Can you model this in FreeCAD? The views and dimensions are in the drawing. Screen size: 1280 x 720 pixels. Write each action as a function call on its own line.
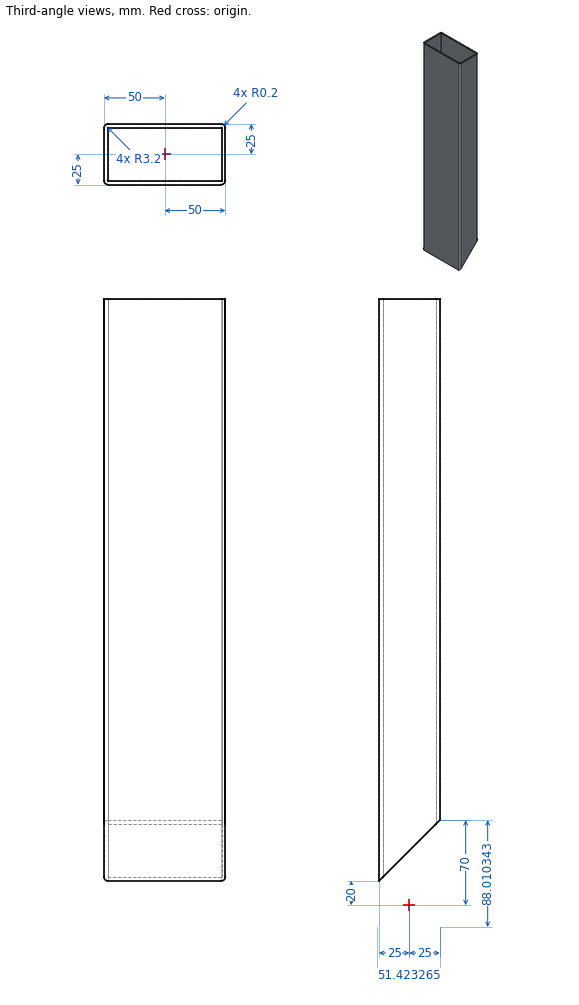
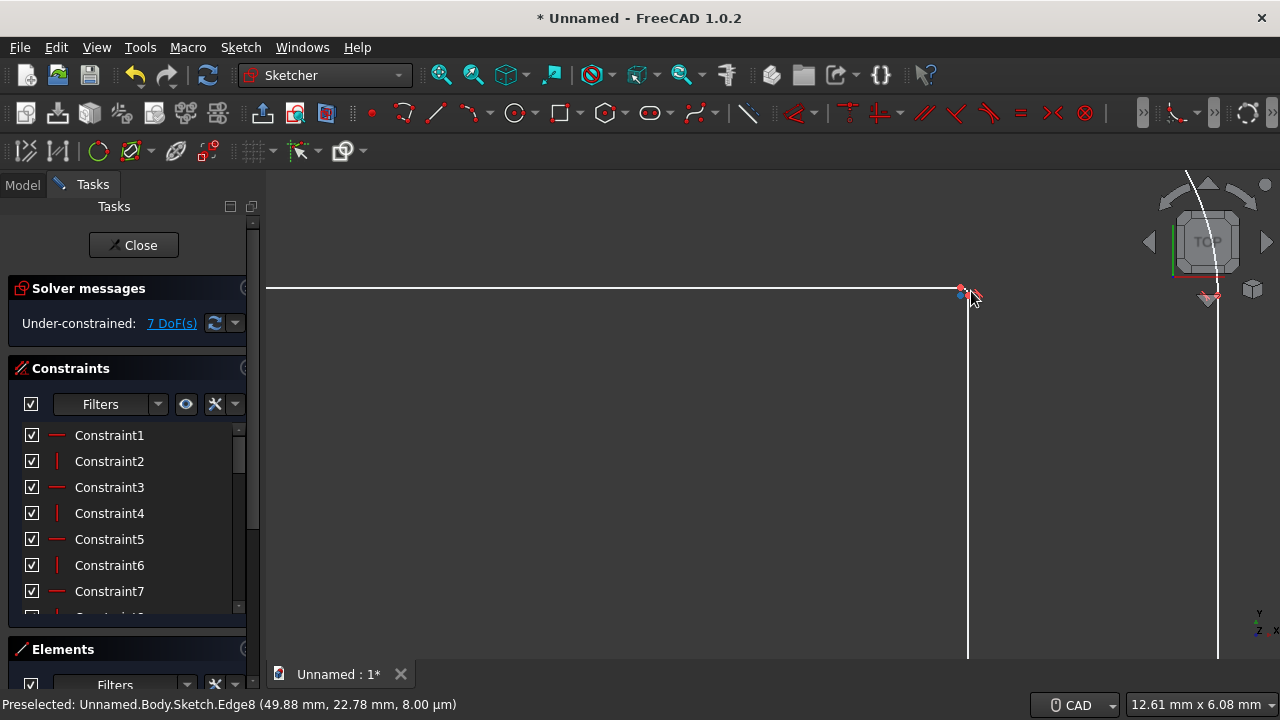
scroll(966, 290, up, 4)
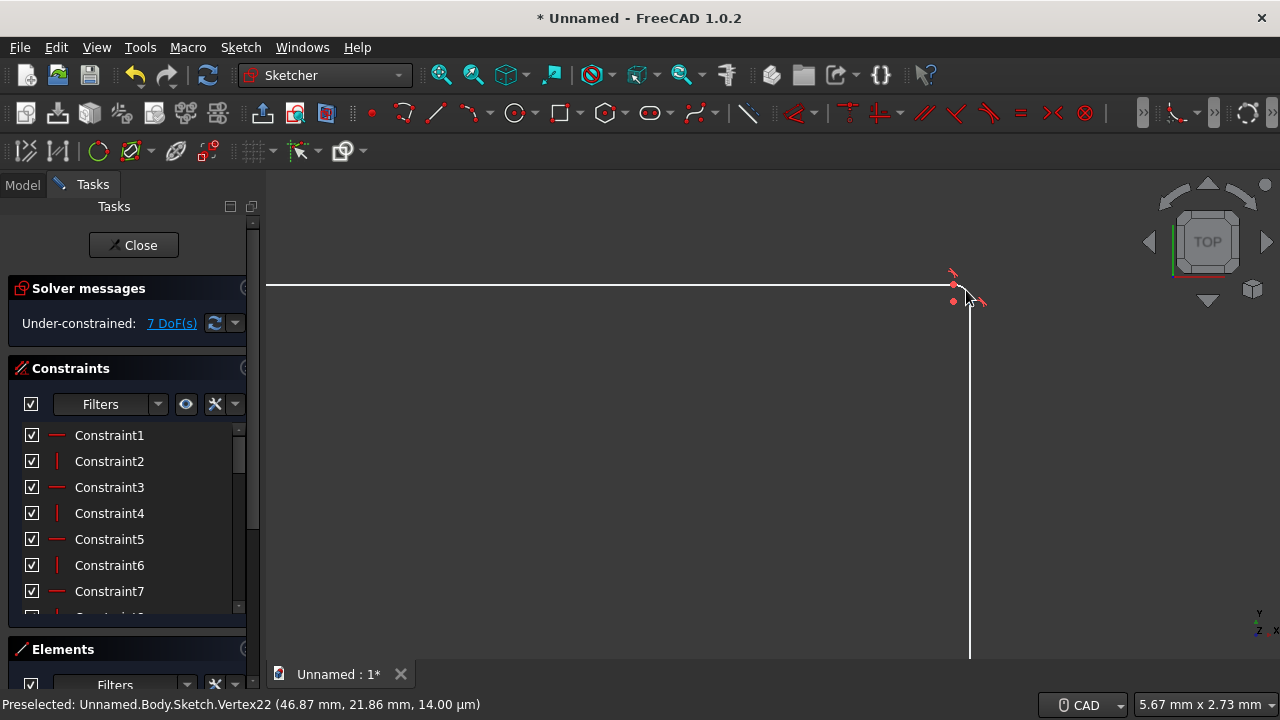
click(965, 290)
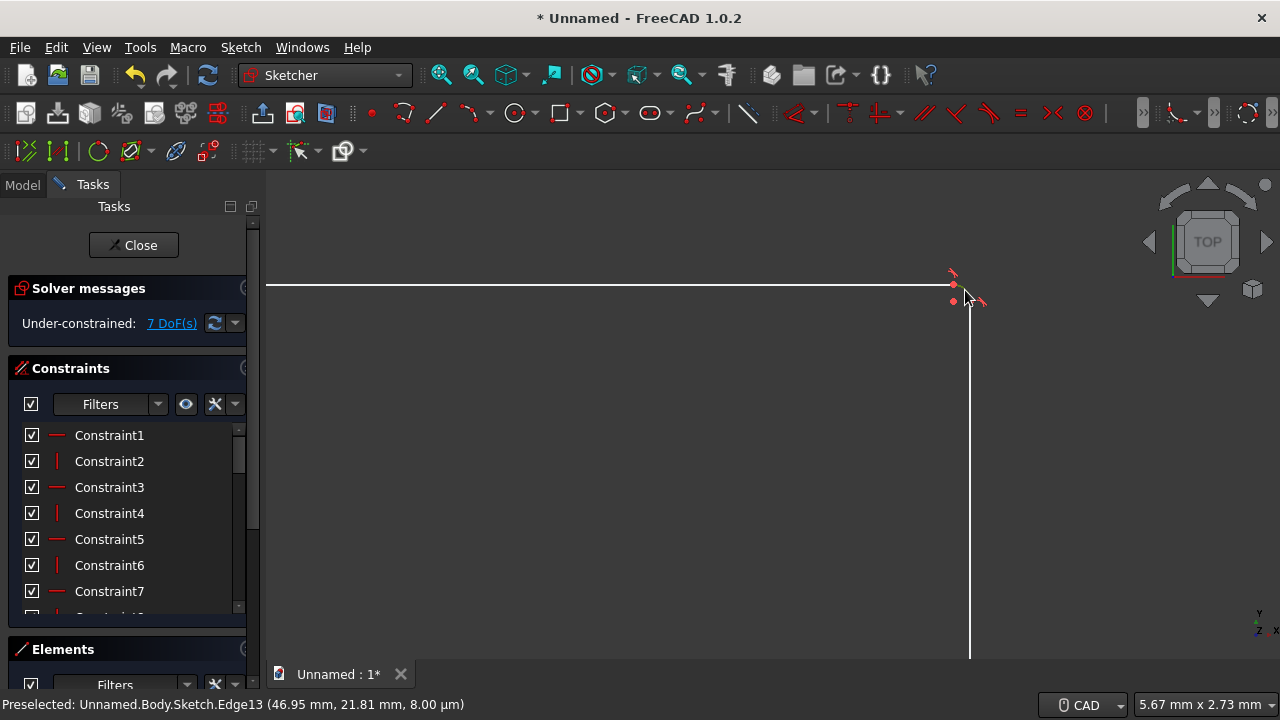
scroll(1050, 254, down, 16)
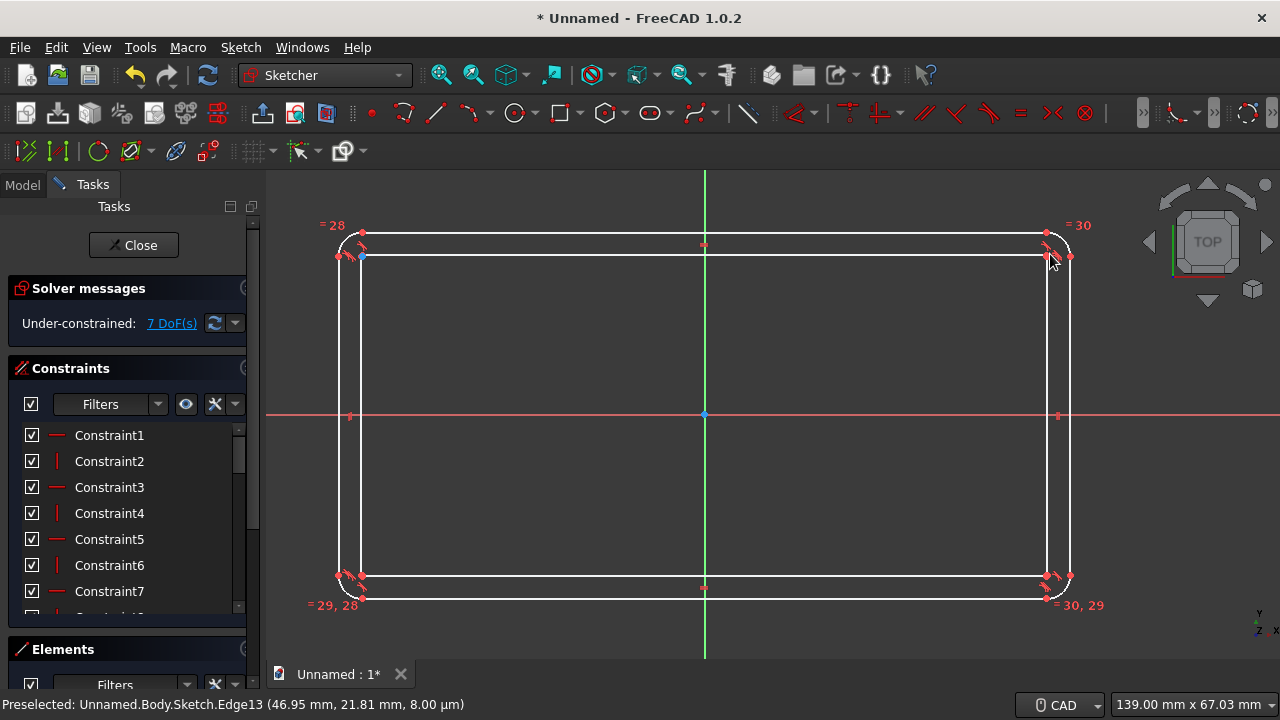
scroll(362, 256, up, 12)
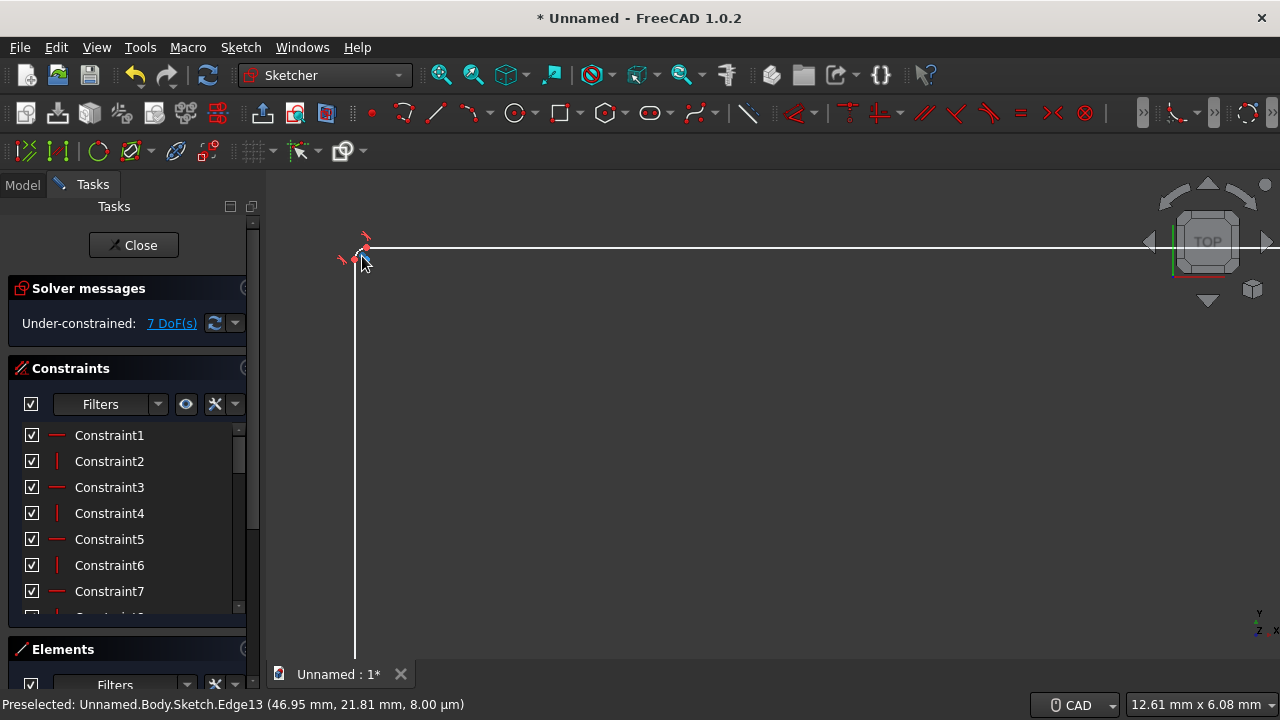
click(361, 249)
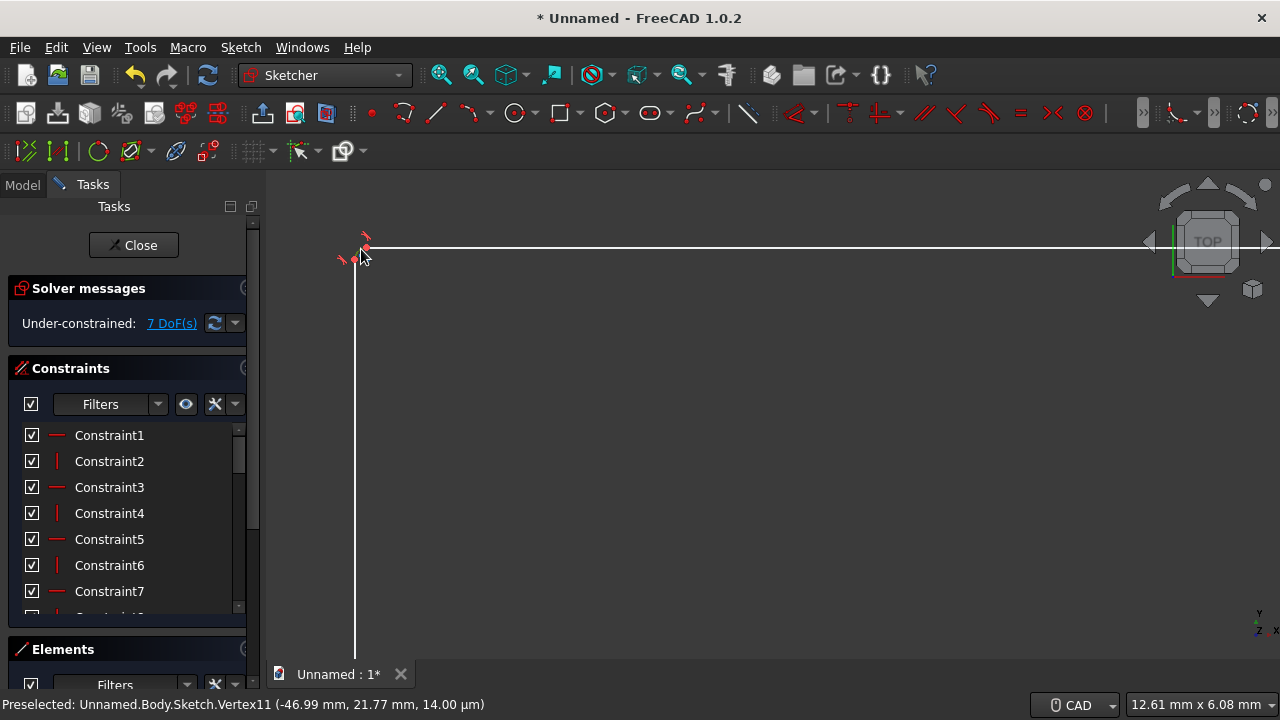
click(1022, 114)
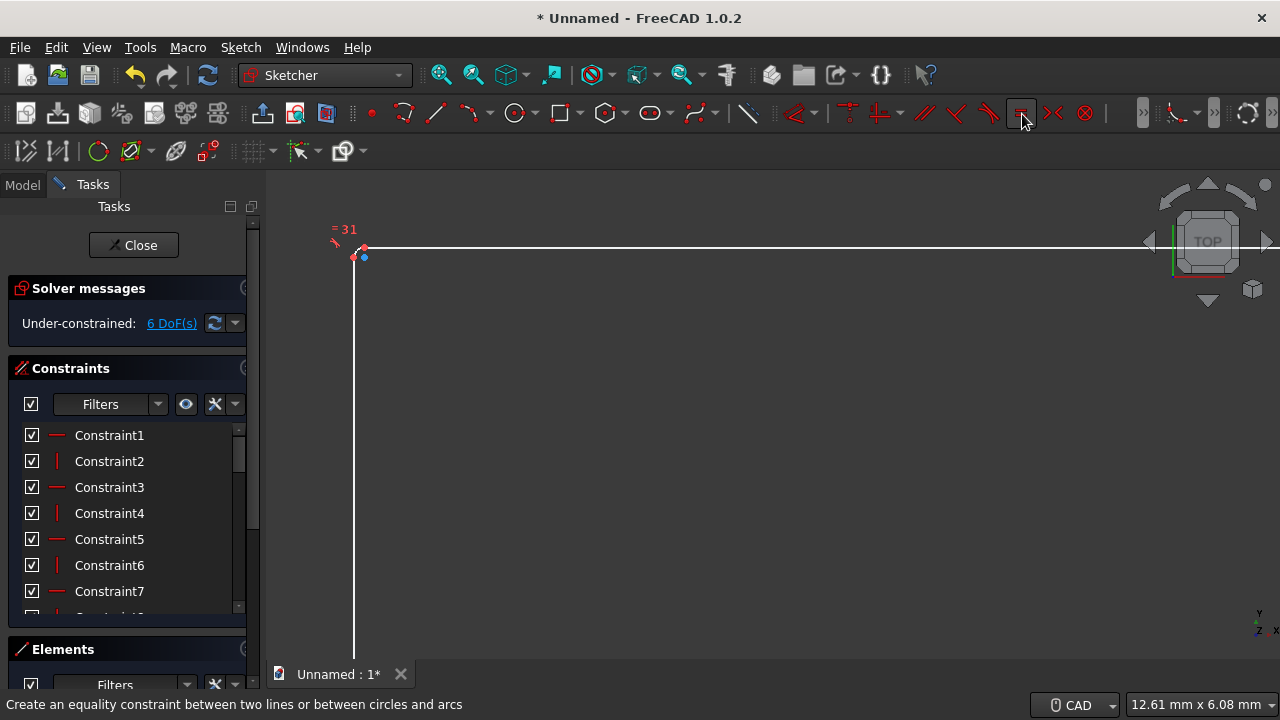
scroll(429, 287, down, 13)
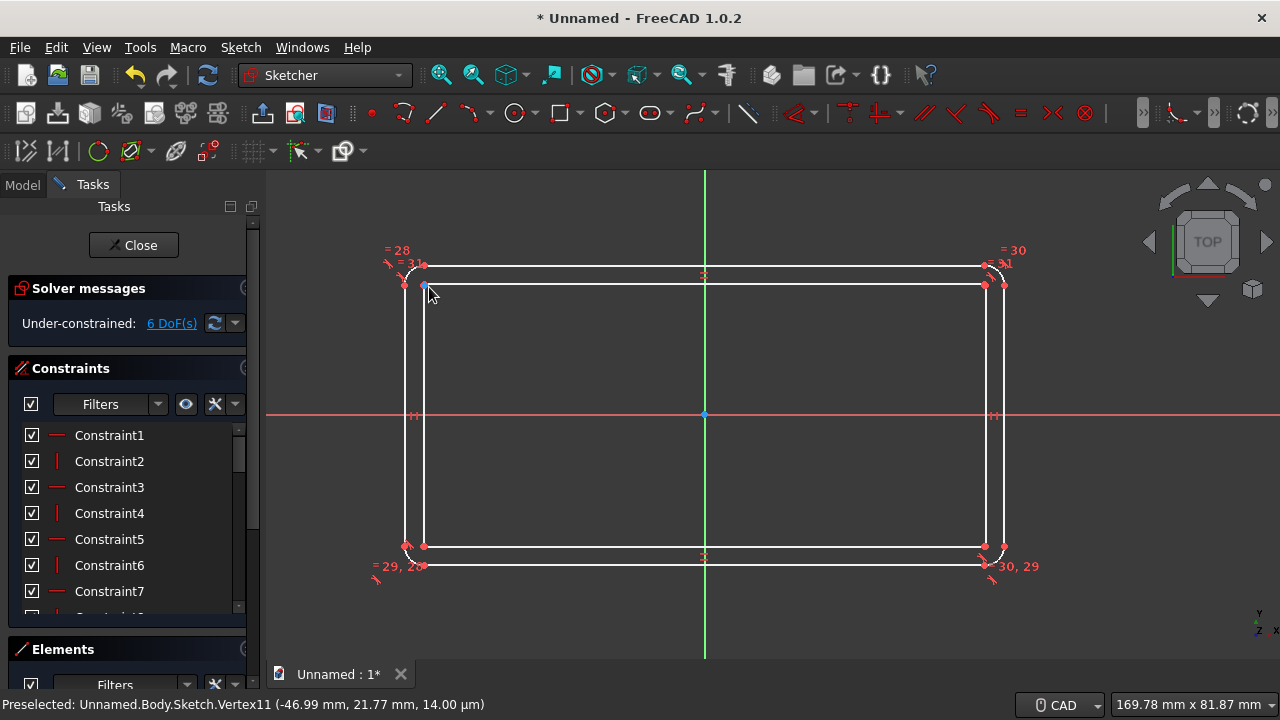
scroll(416, 268, up, 4)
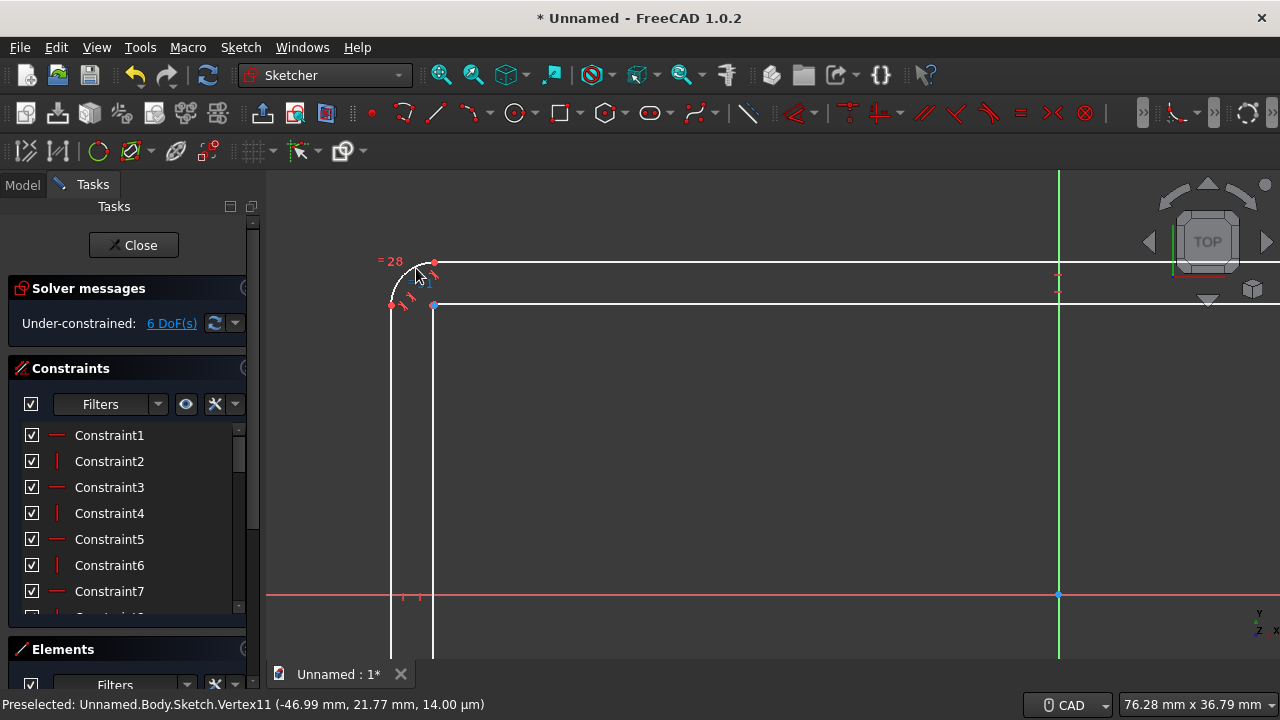
click(415, 267)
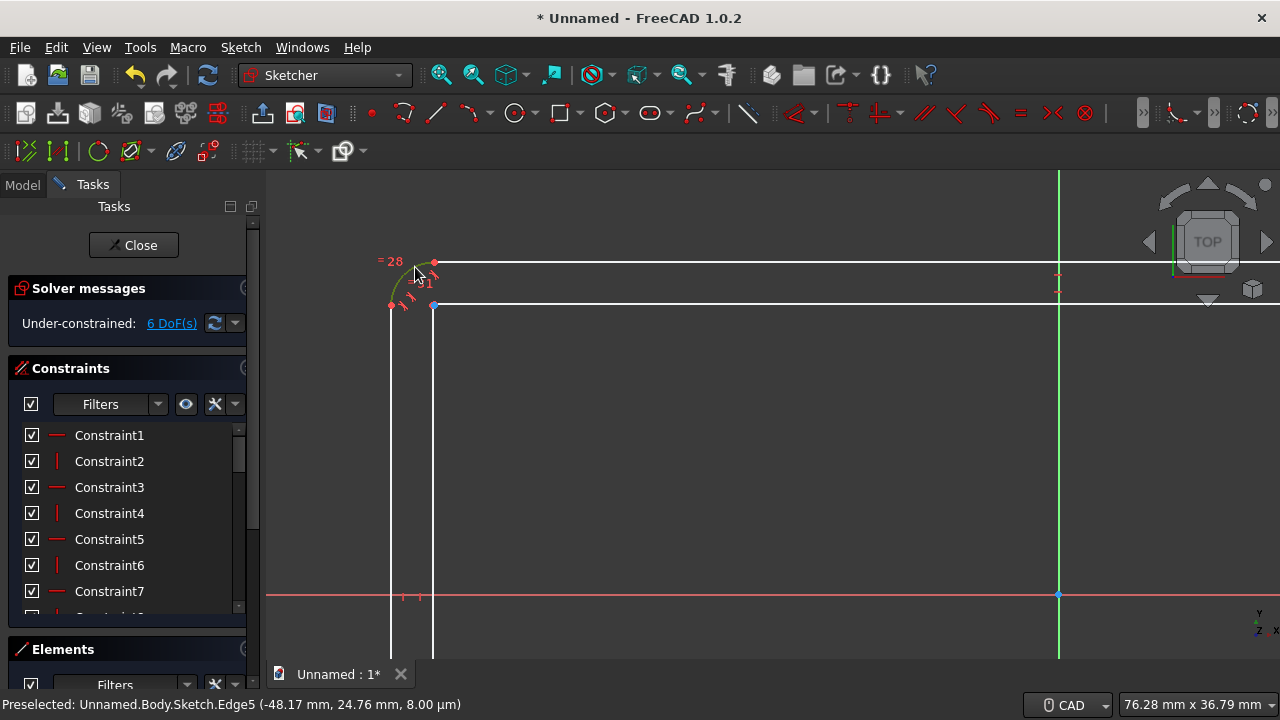
click(816, 114)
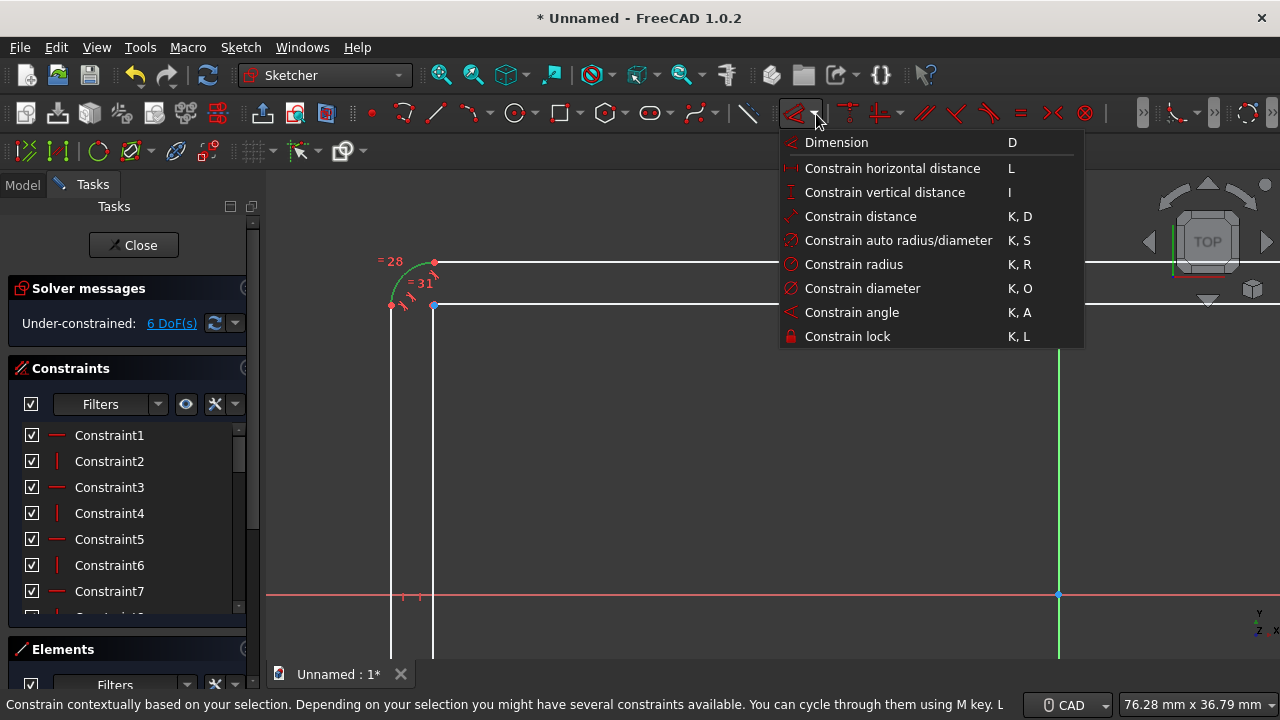
click(932, 264)